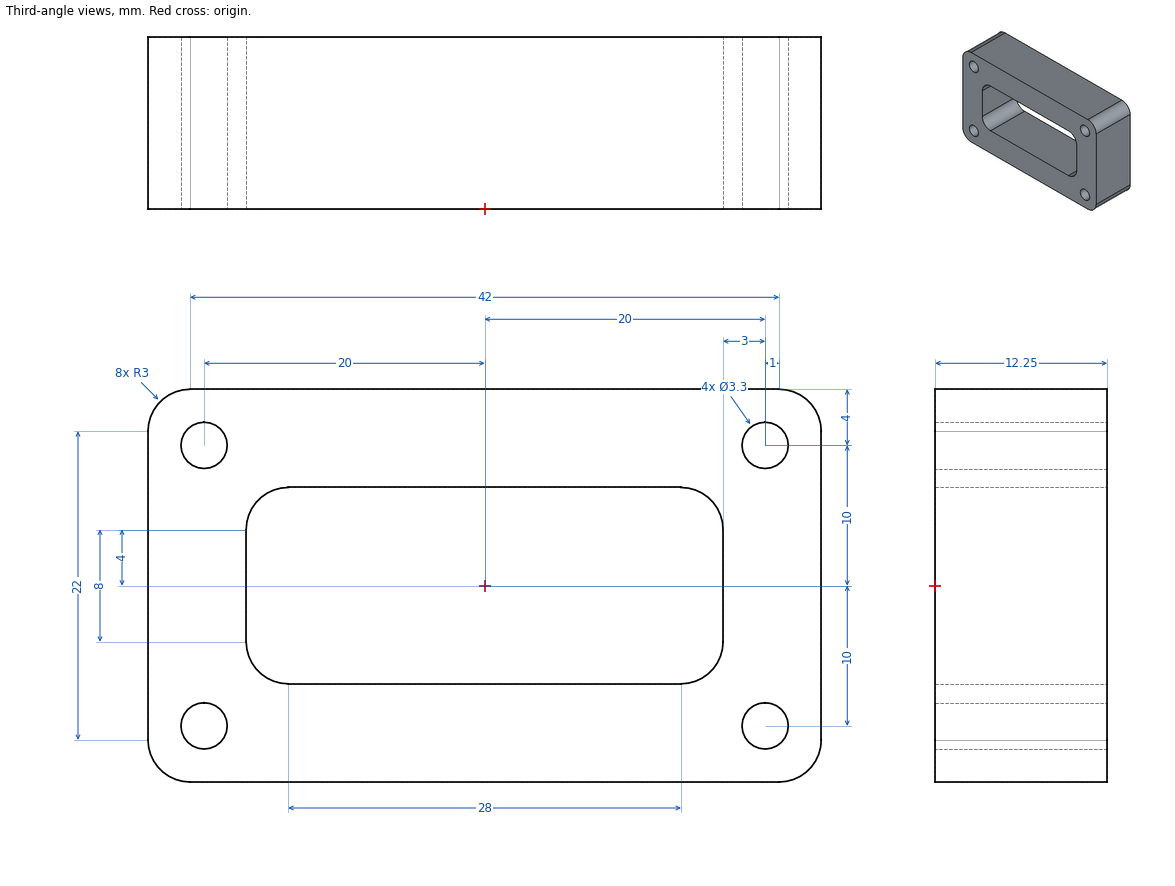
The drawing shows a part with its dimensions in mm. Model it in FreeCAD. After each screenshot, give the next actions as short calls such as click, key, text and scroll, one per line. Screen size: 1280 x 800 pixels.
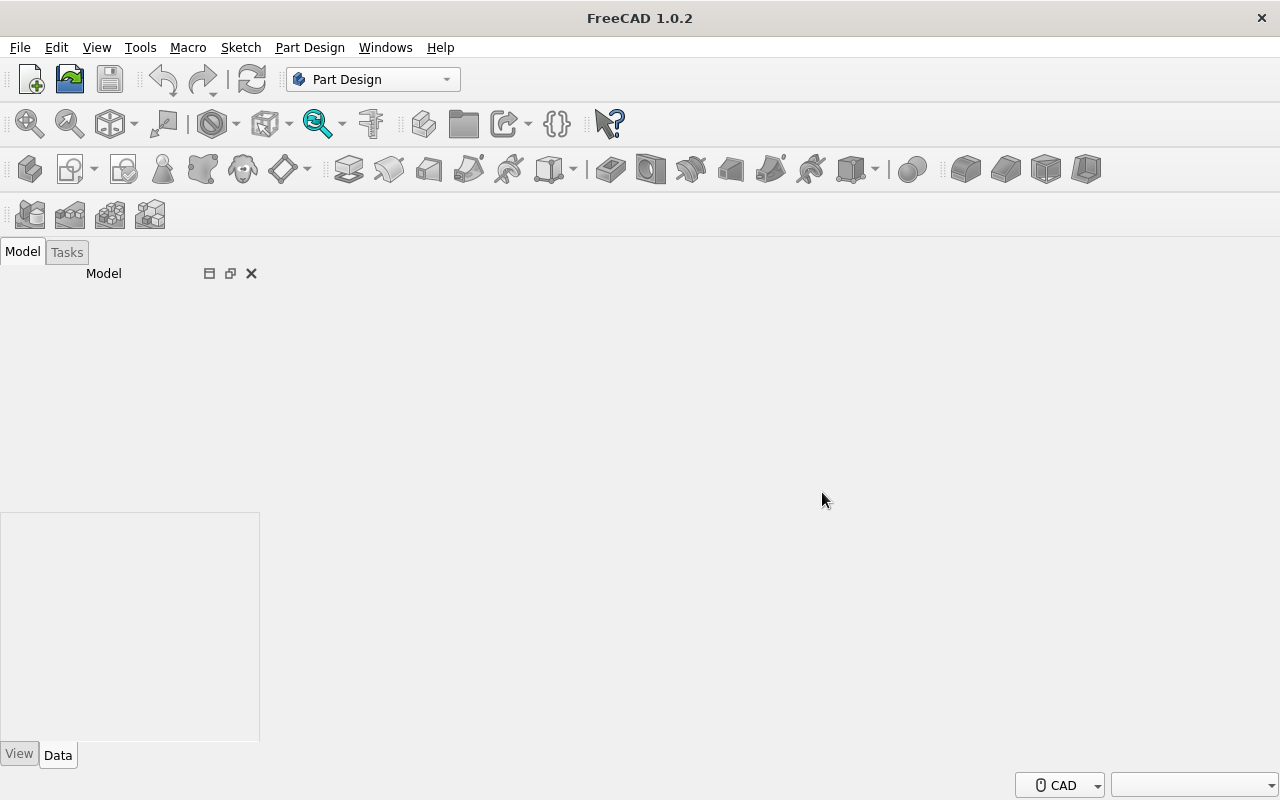
click(30, 80)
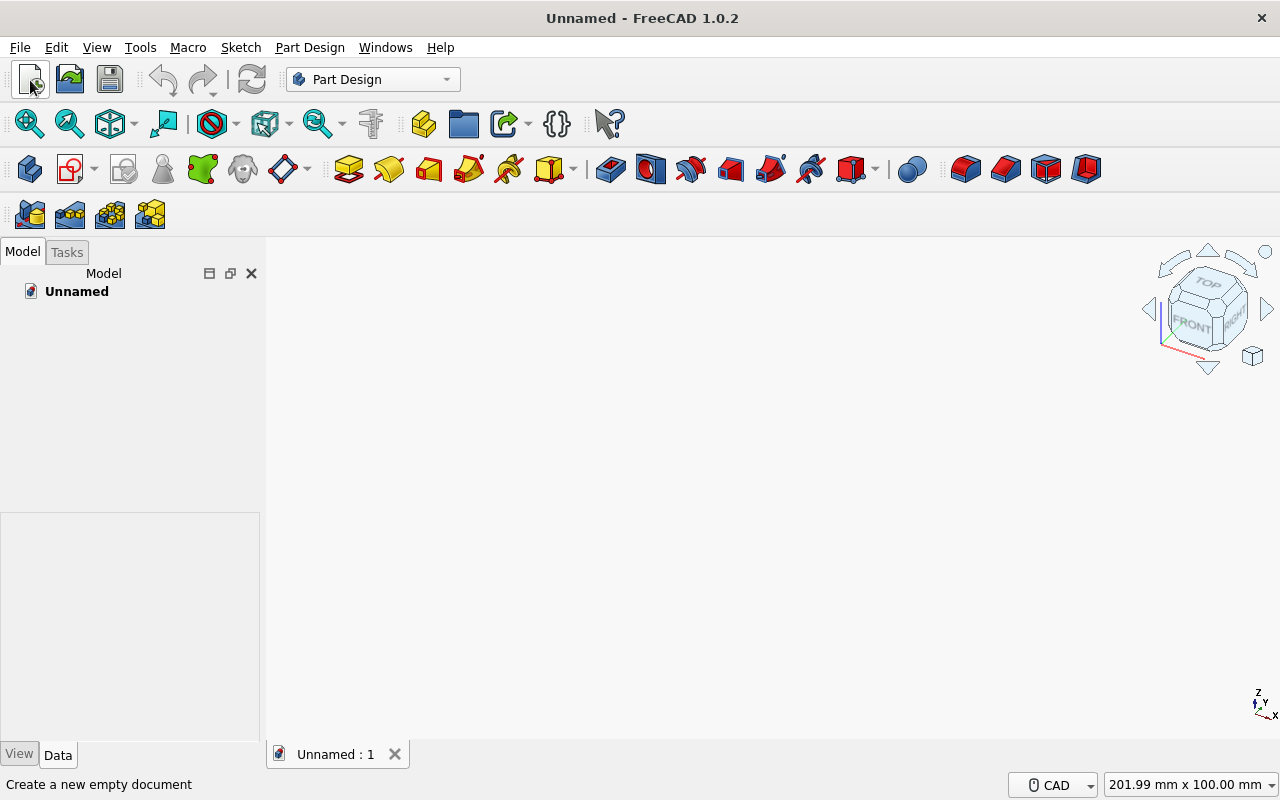
click(70, 170)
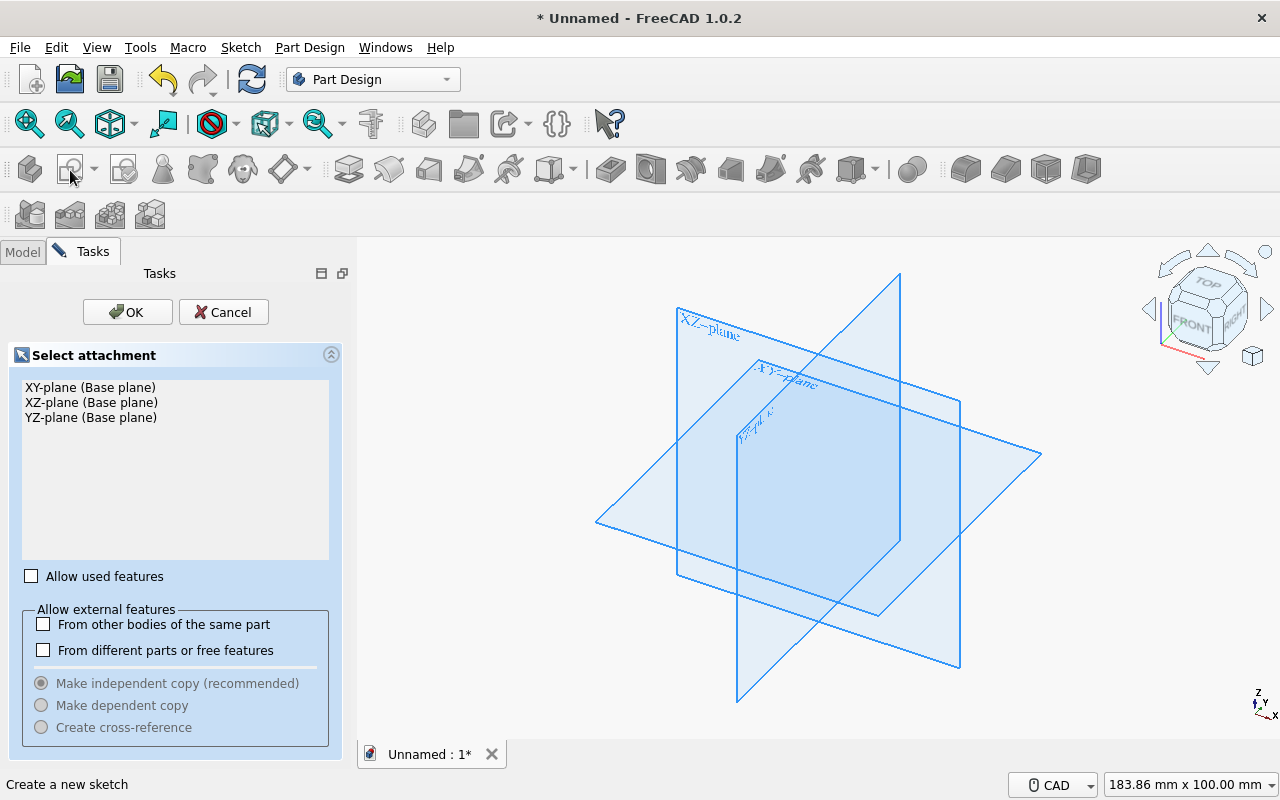
click(82, 402)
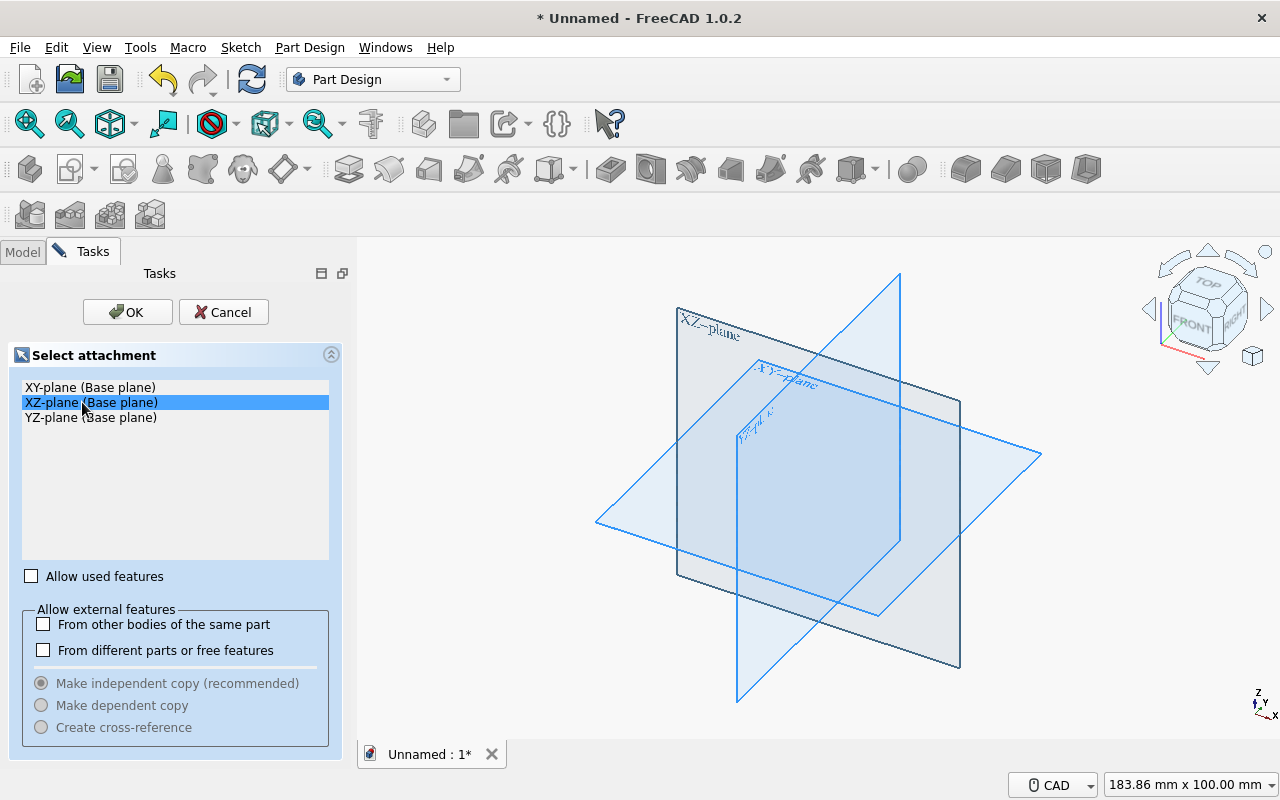
click(128, 312)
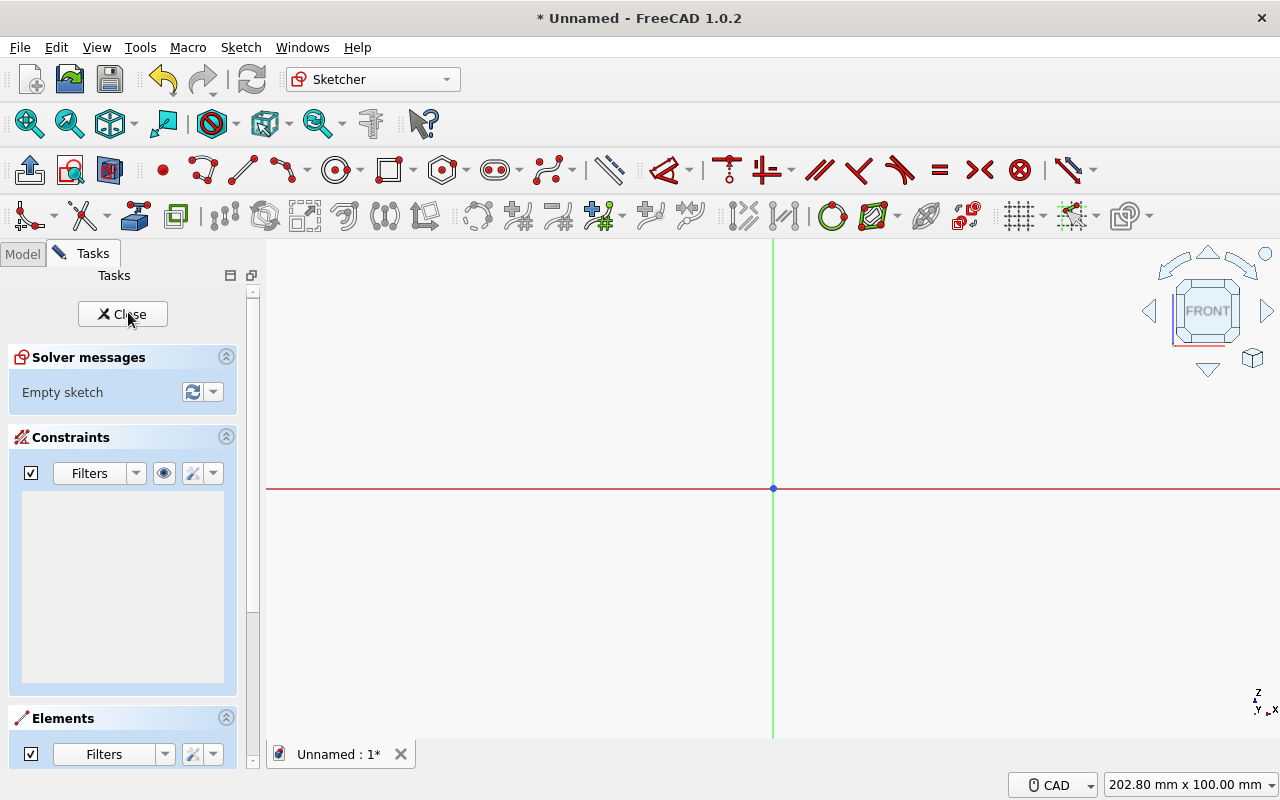
scroll(829, 489, up, 4)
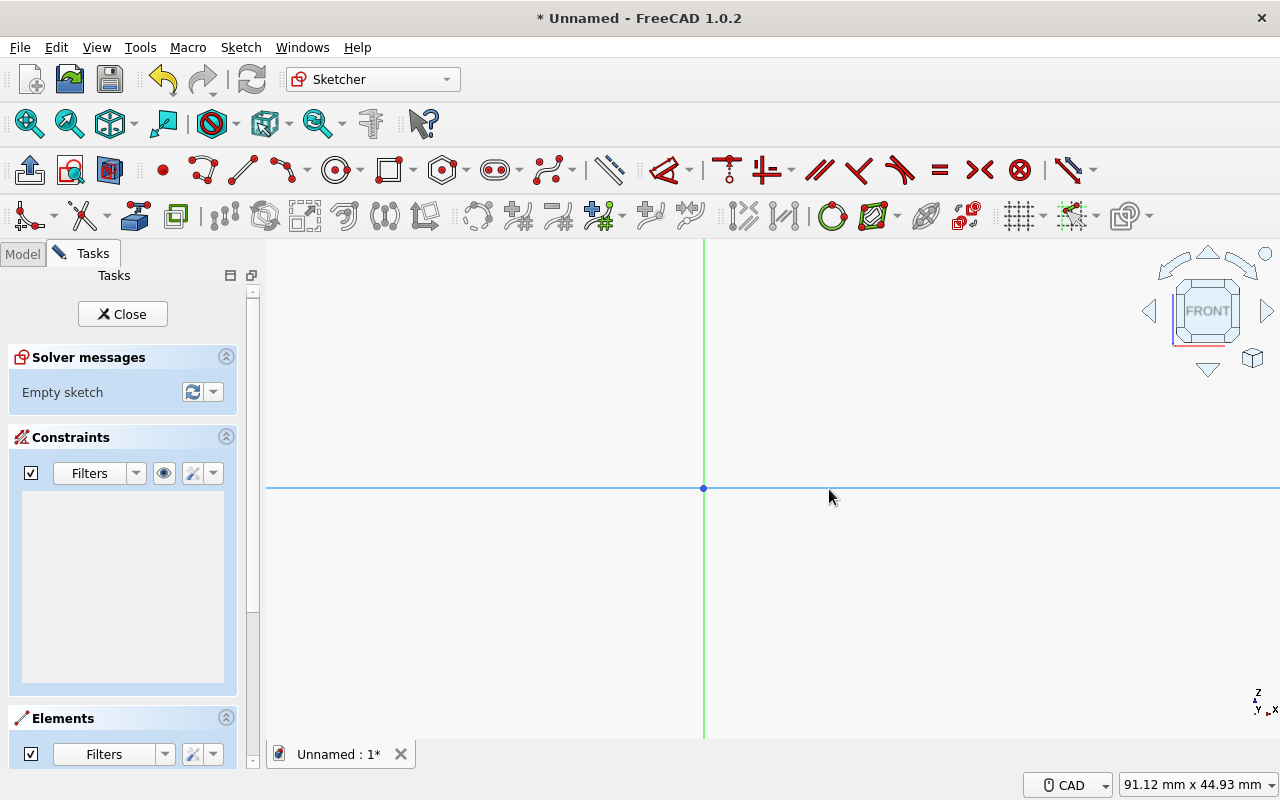
click(244, 170)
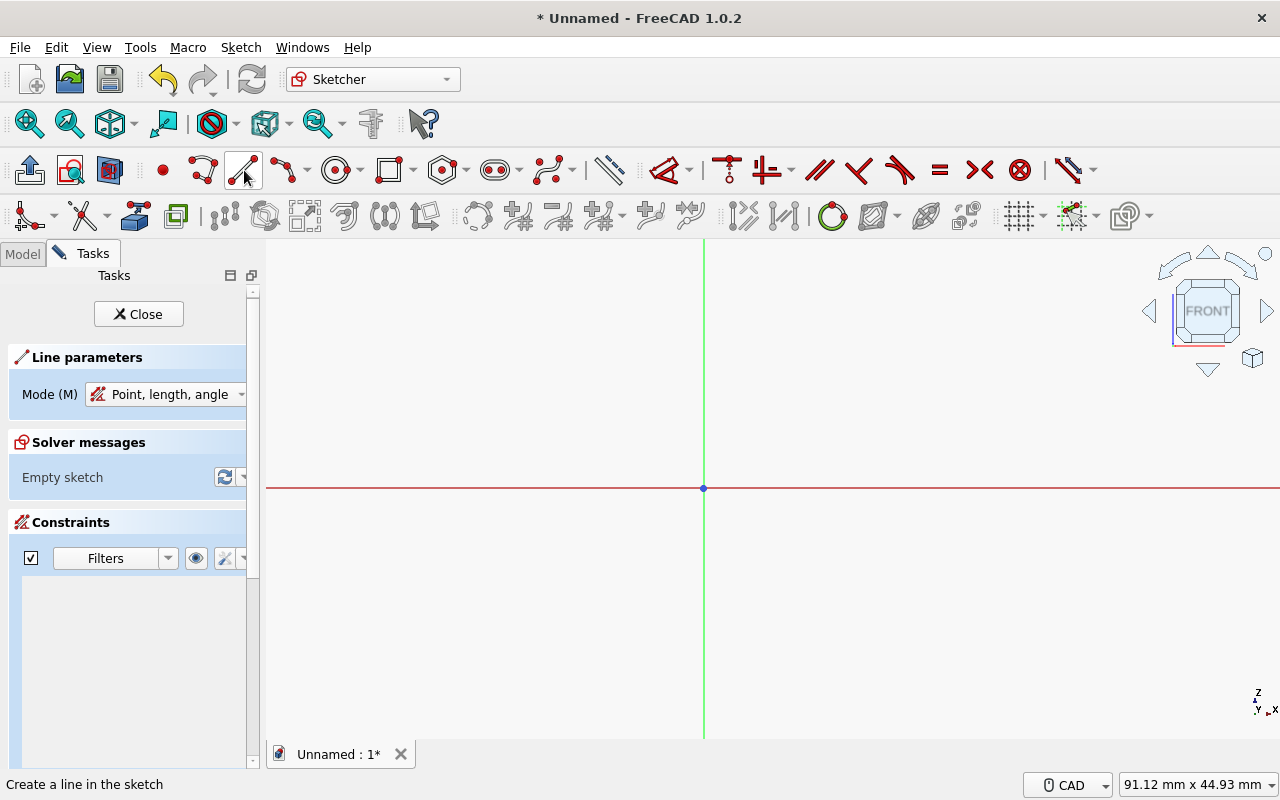
click(437, 611)
click(437, 366)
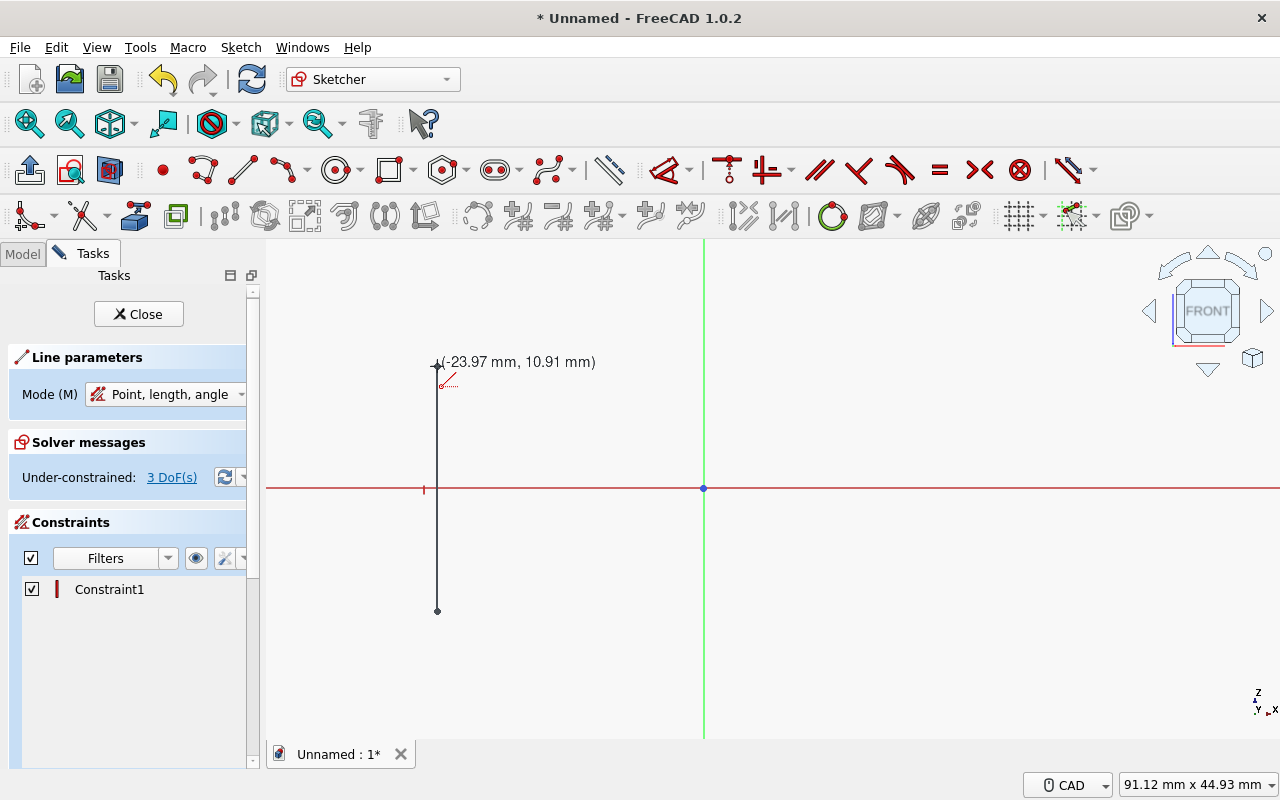
click(470, 333)
click(937, 333)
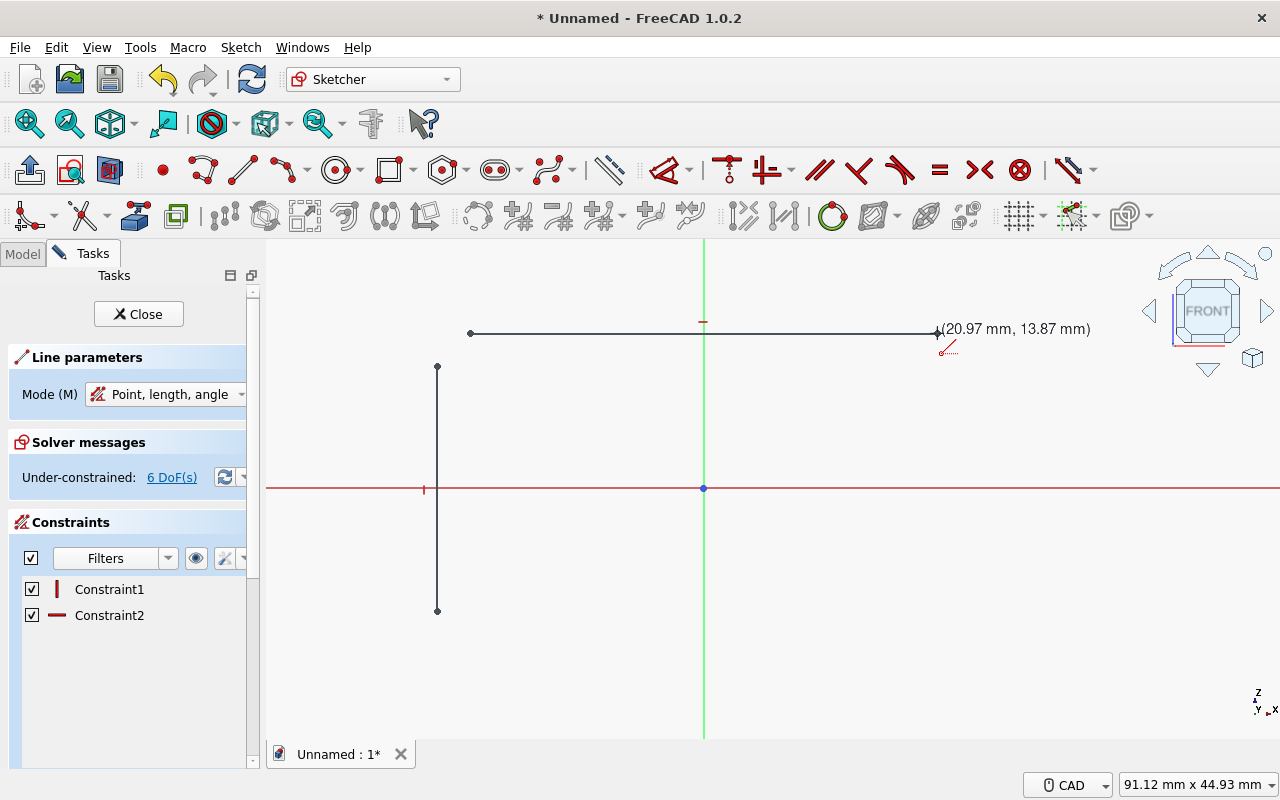
click(971, 366)
click(971, 611)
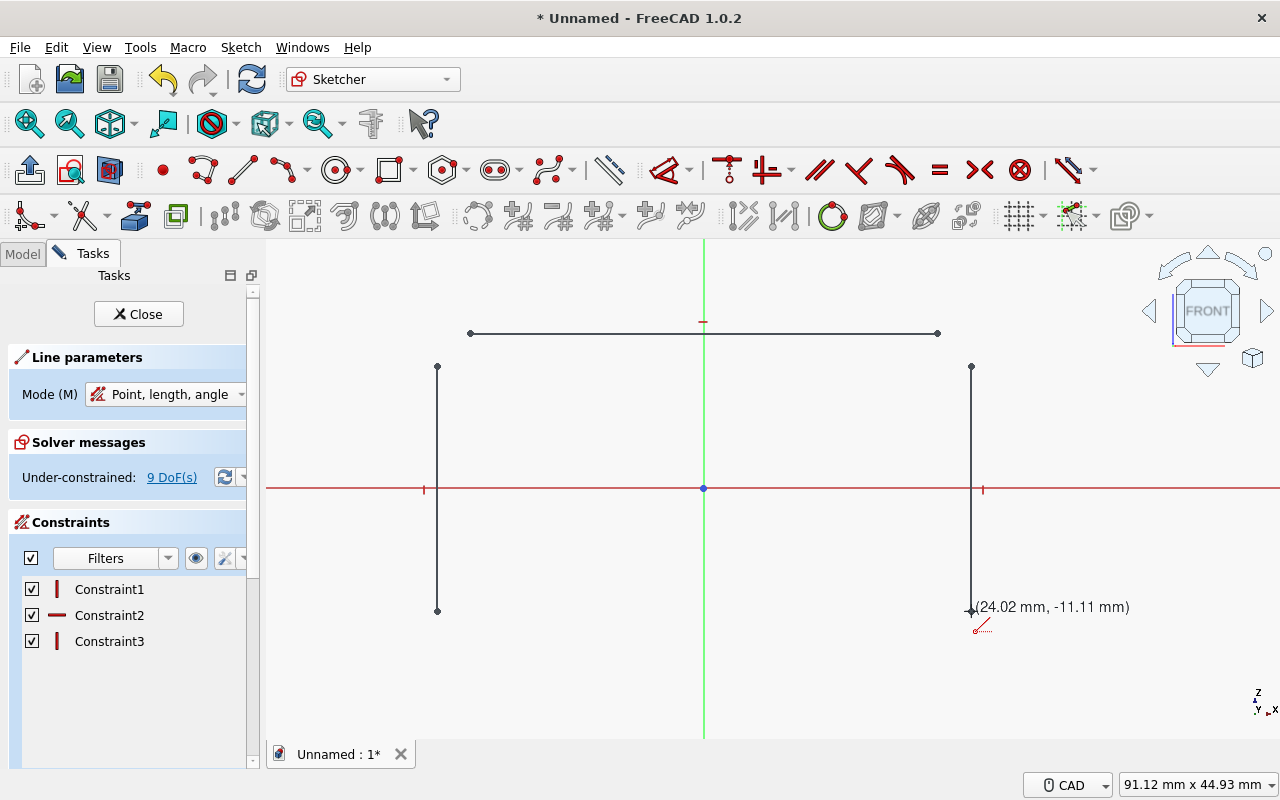
click(937, 644)
click(470, 644)